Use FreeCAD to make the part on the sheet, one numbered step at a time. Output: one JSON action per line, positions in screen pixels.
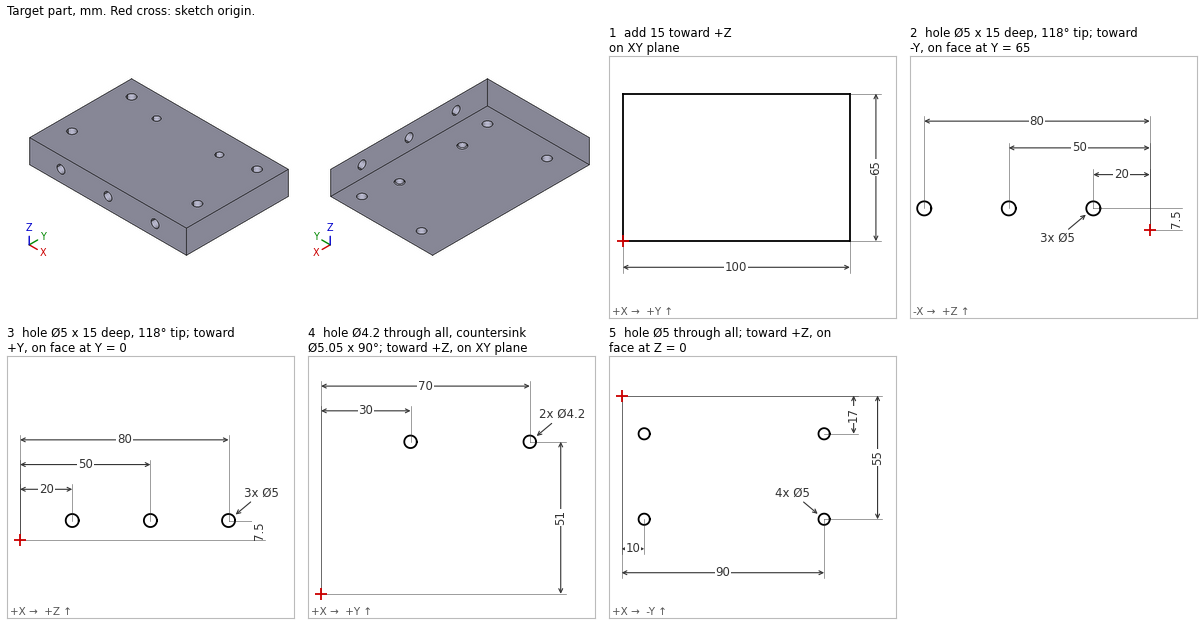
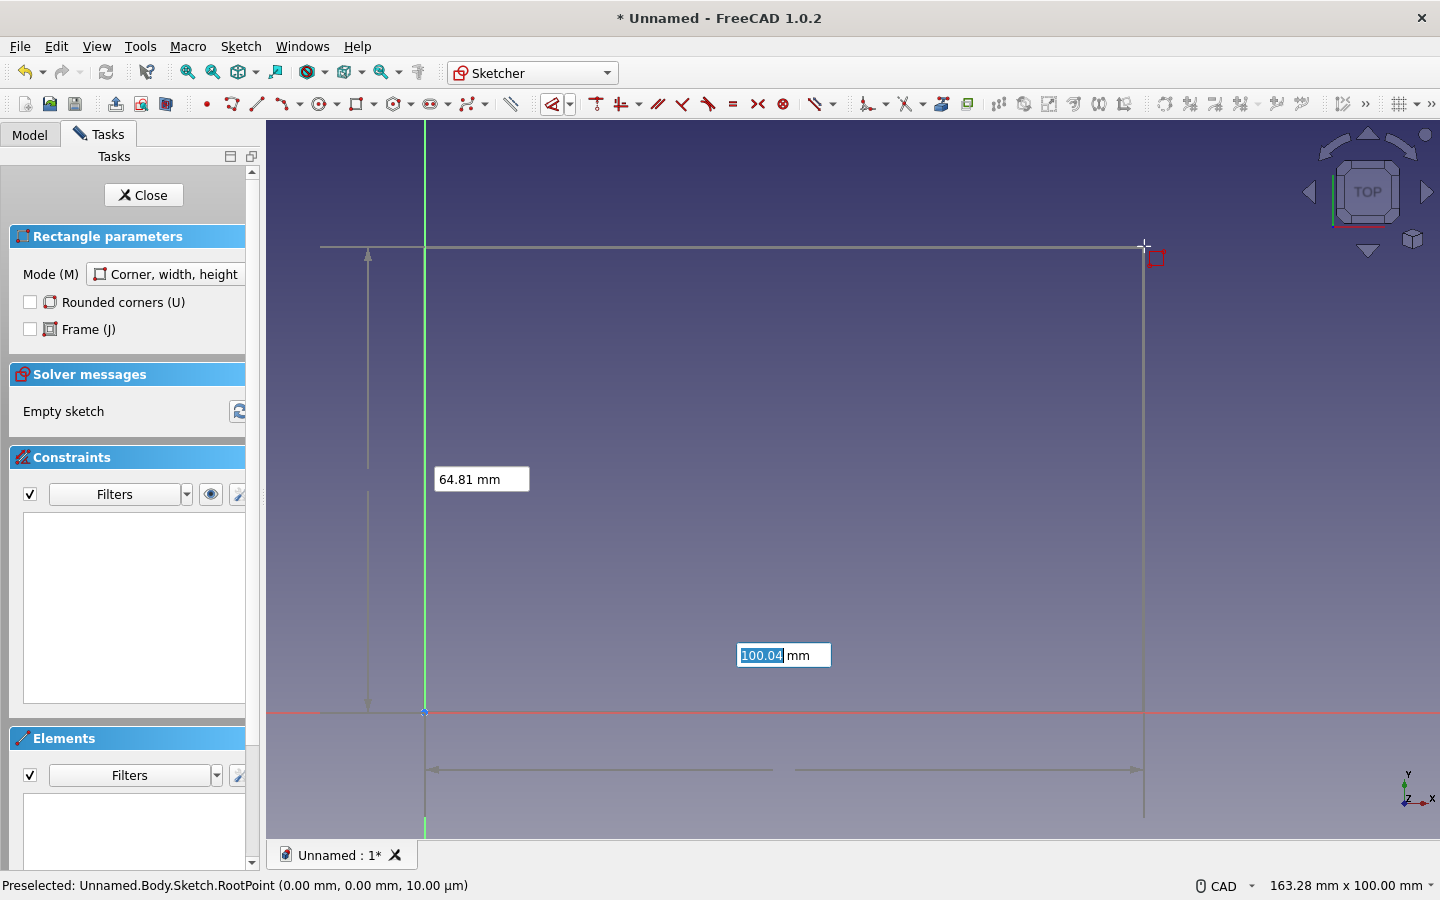
{"action": "type", "text": "100"}
{"action": "key", "text": "Tab"}
{"action": "type", "text": "65"}
{"action": "key", "text": "Return"}
{"action": "key", "text": "Escape"}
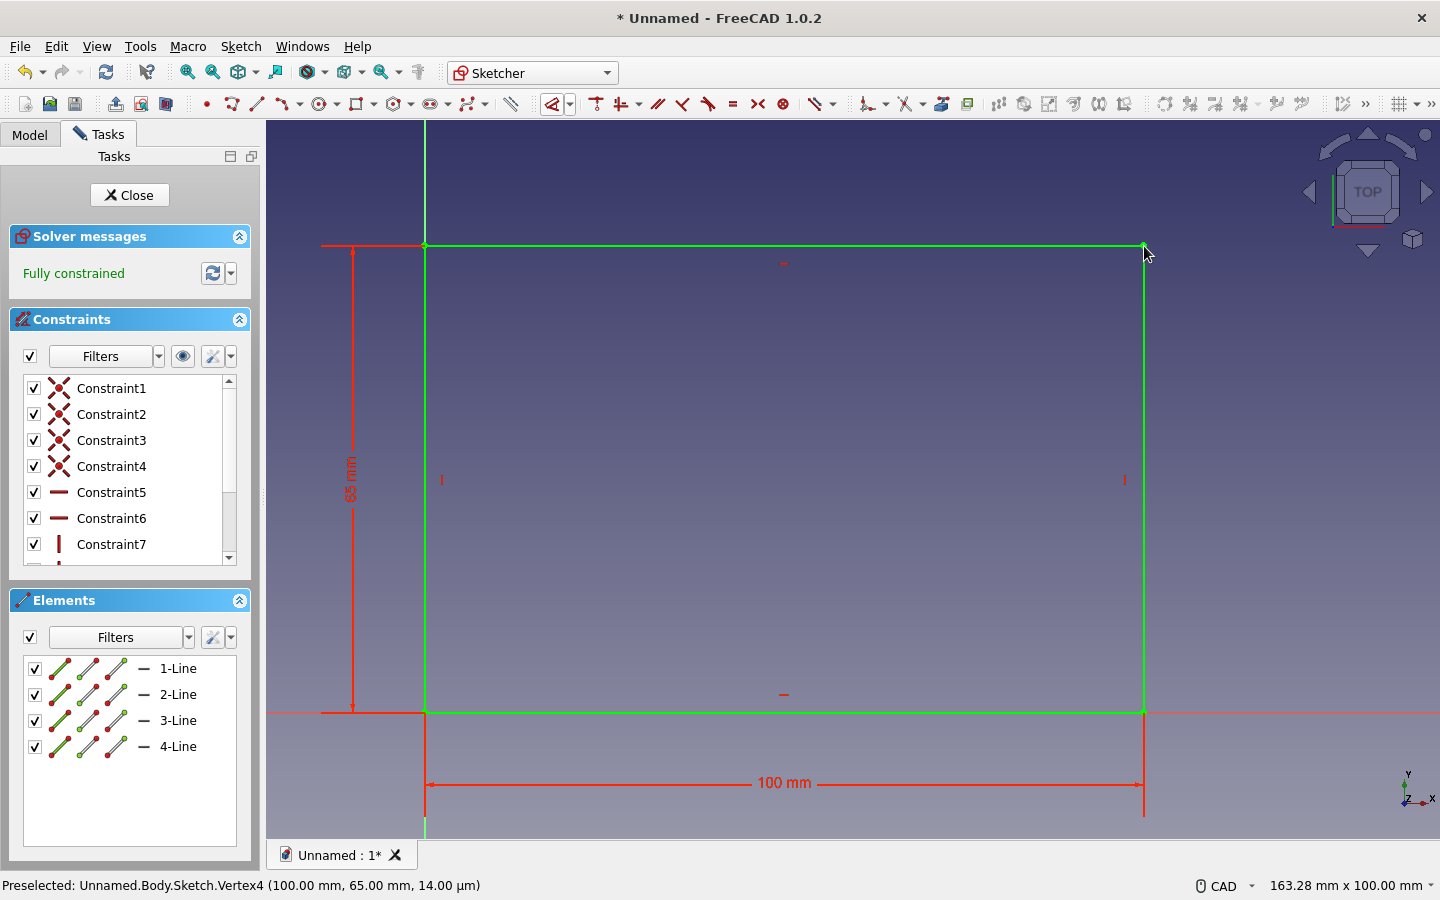
{"action": "left_click", "coordinate": [130, 195]}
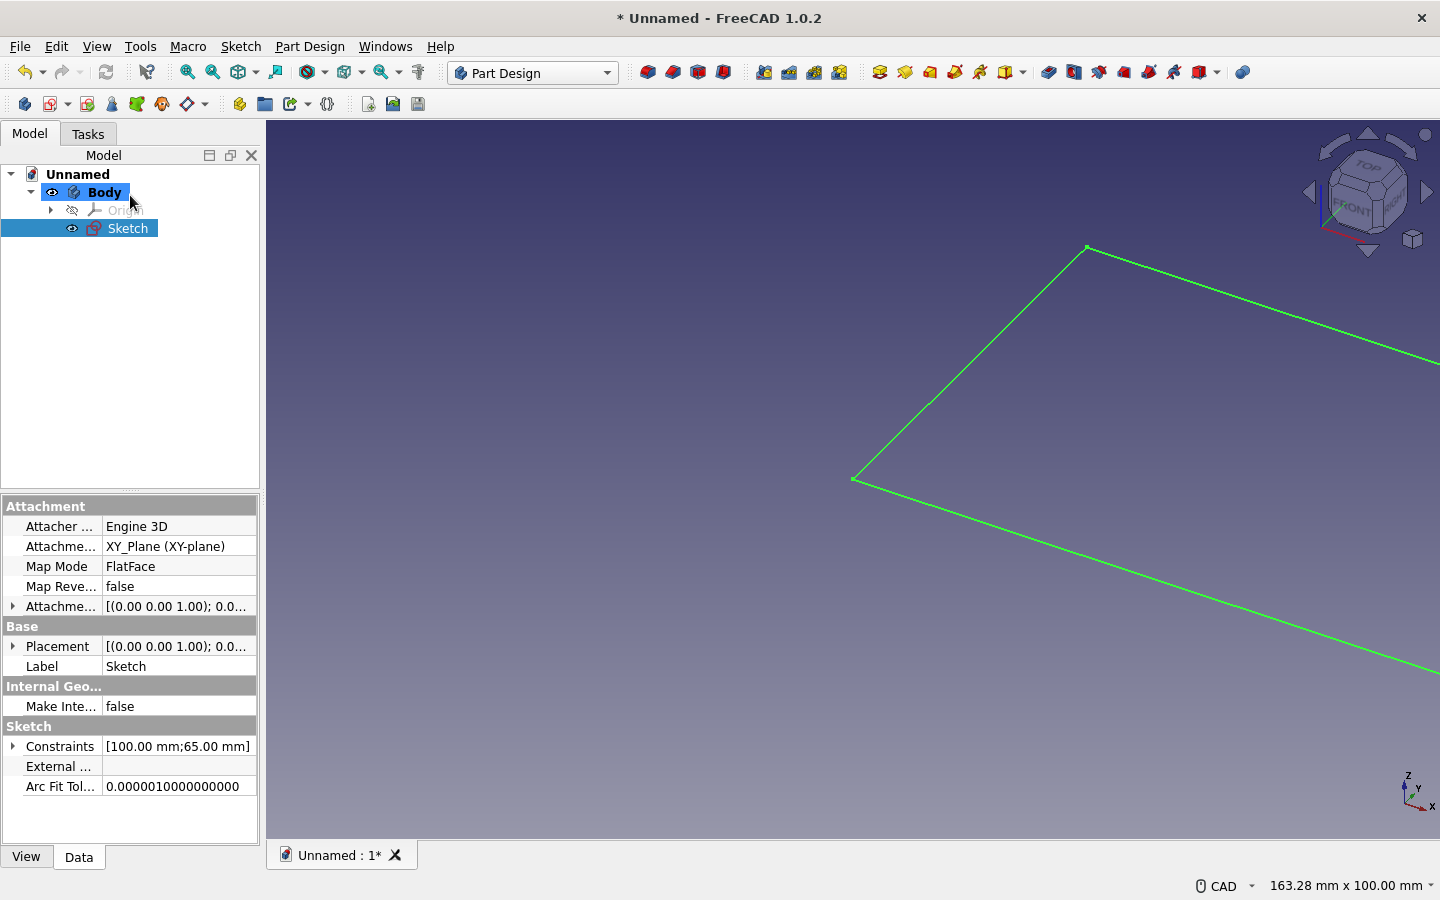
{"action": "left_click", "coordinate": [880, 72]}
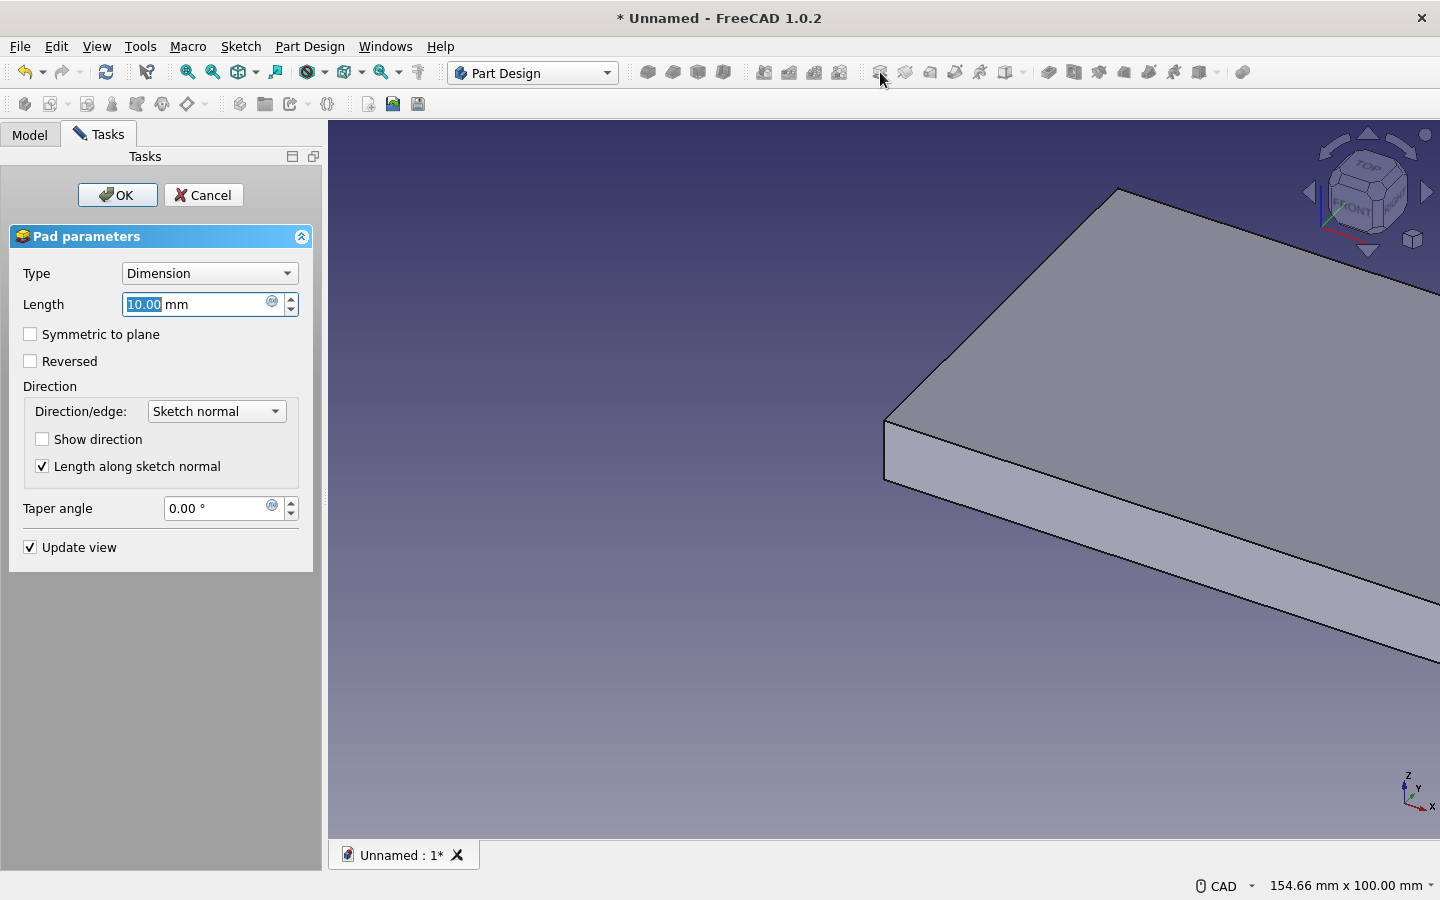
{"action": "type", "text": "15"}
{"action": "key", "text": "Tab"}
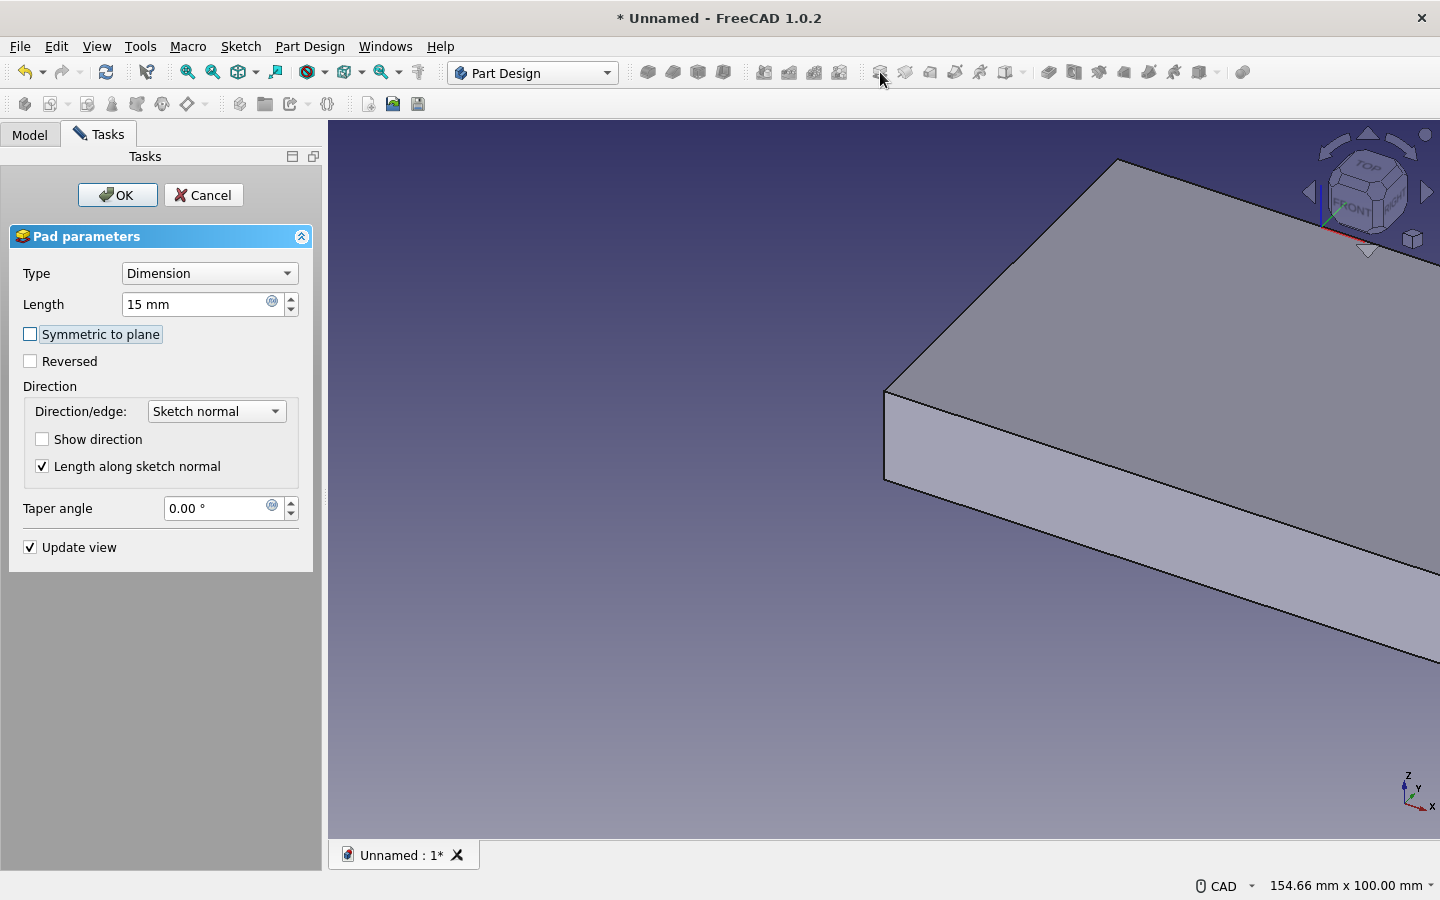
{"action": "left_click", "coordinate": [118, 195]}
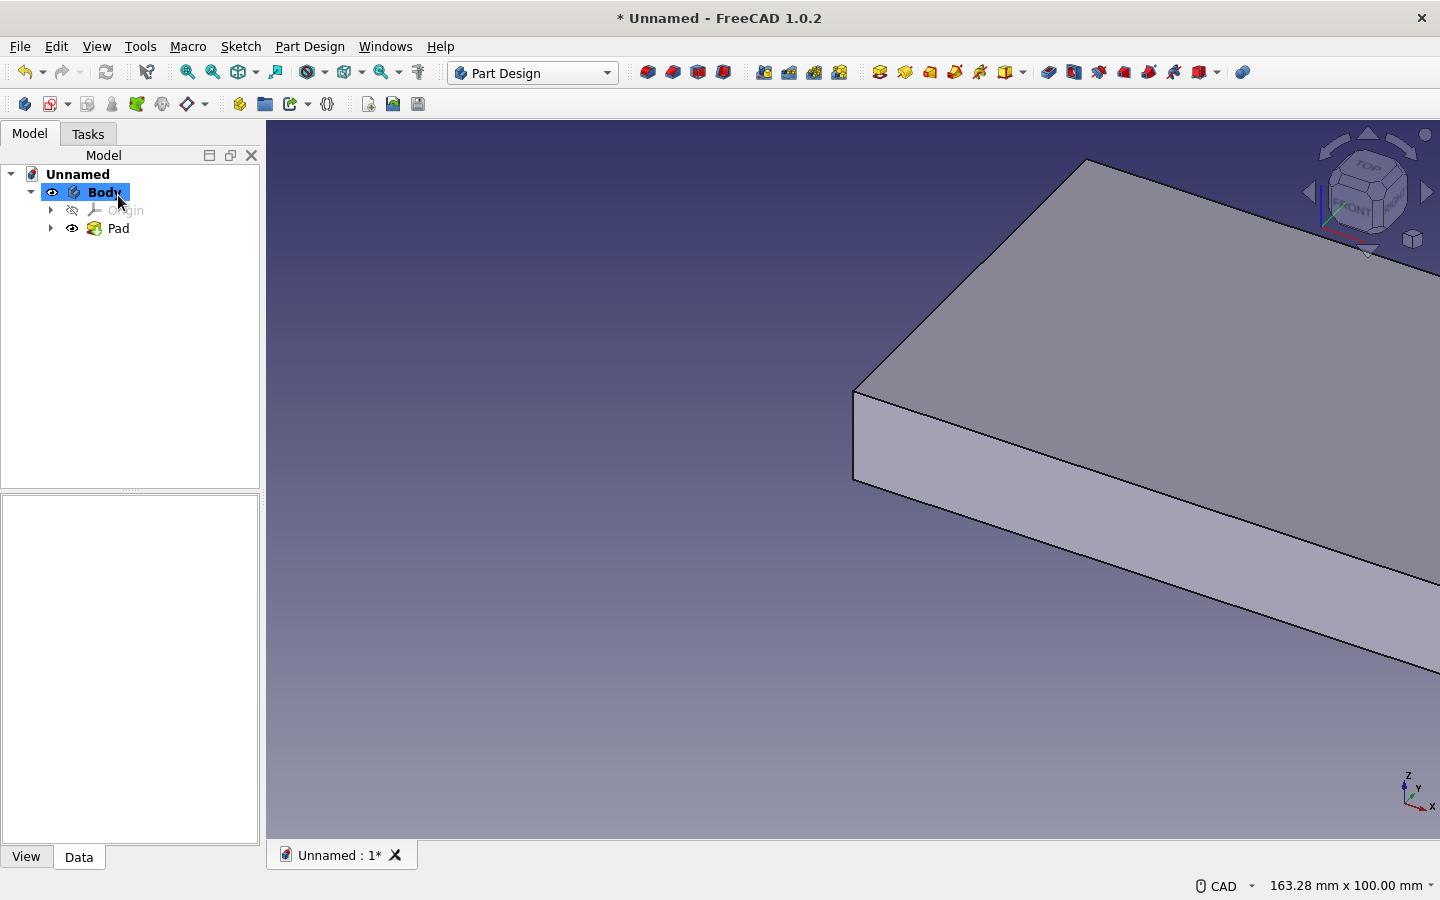
{"action": "left_click", "coordinate": [188, 72]}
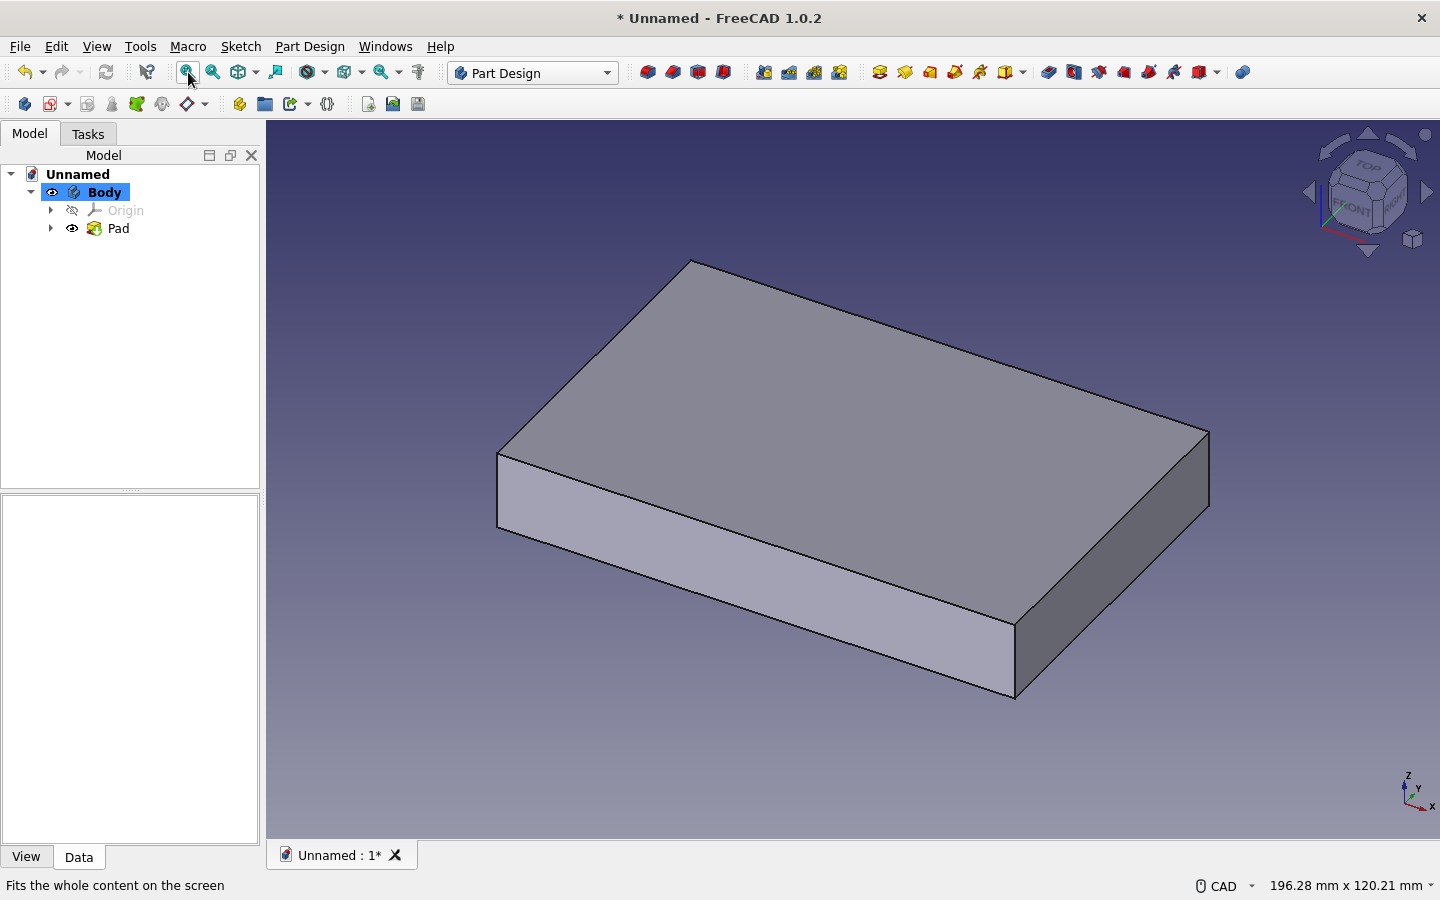
{"action": "key", "text": "4"}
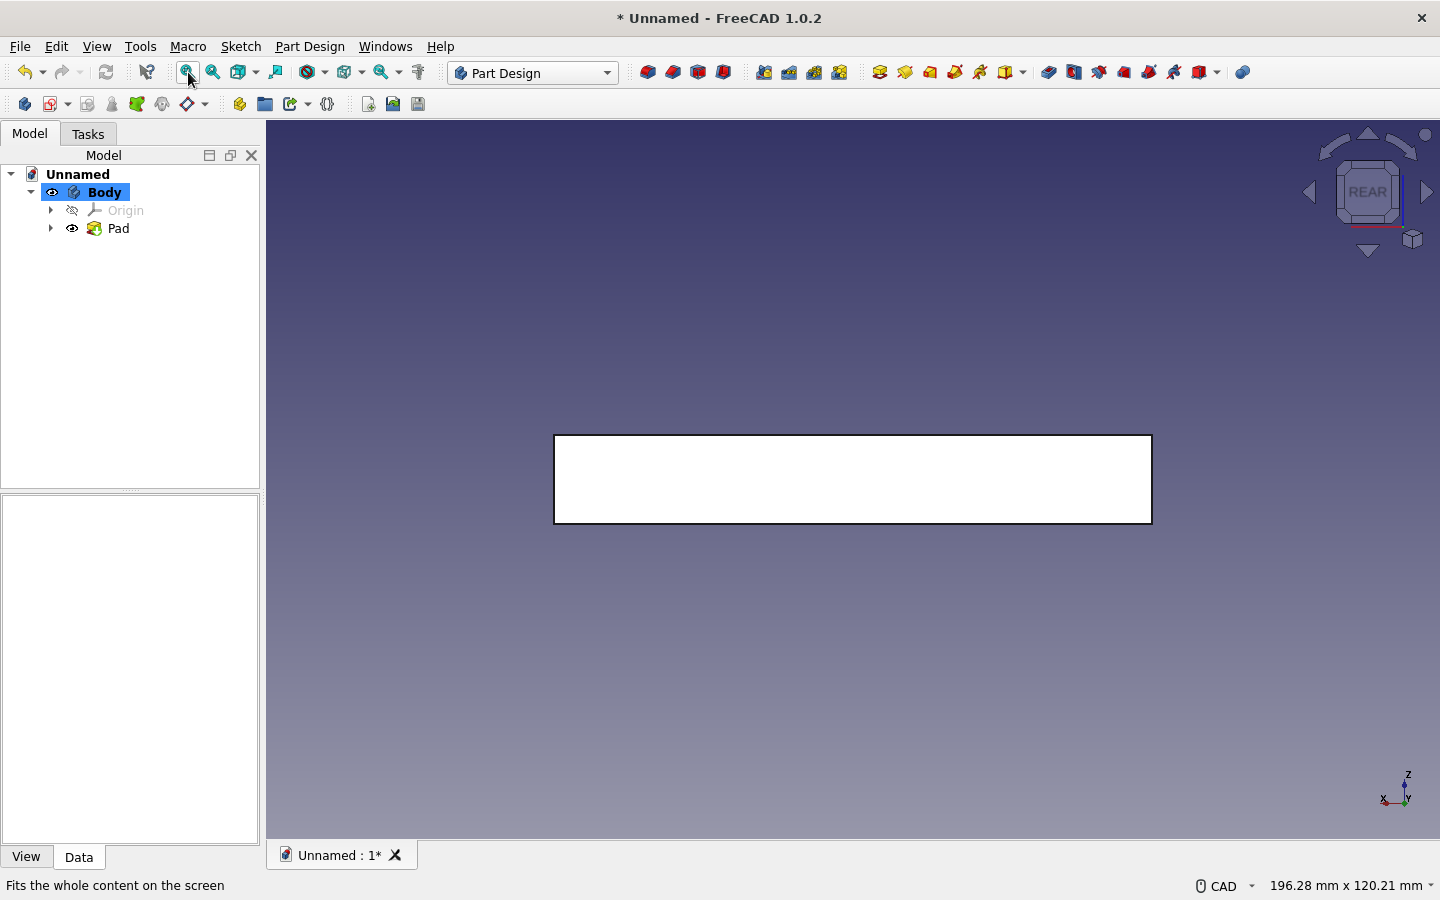
{"action": "left_click", "coordinate": [682, 478]}